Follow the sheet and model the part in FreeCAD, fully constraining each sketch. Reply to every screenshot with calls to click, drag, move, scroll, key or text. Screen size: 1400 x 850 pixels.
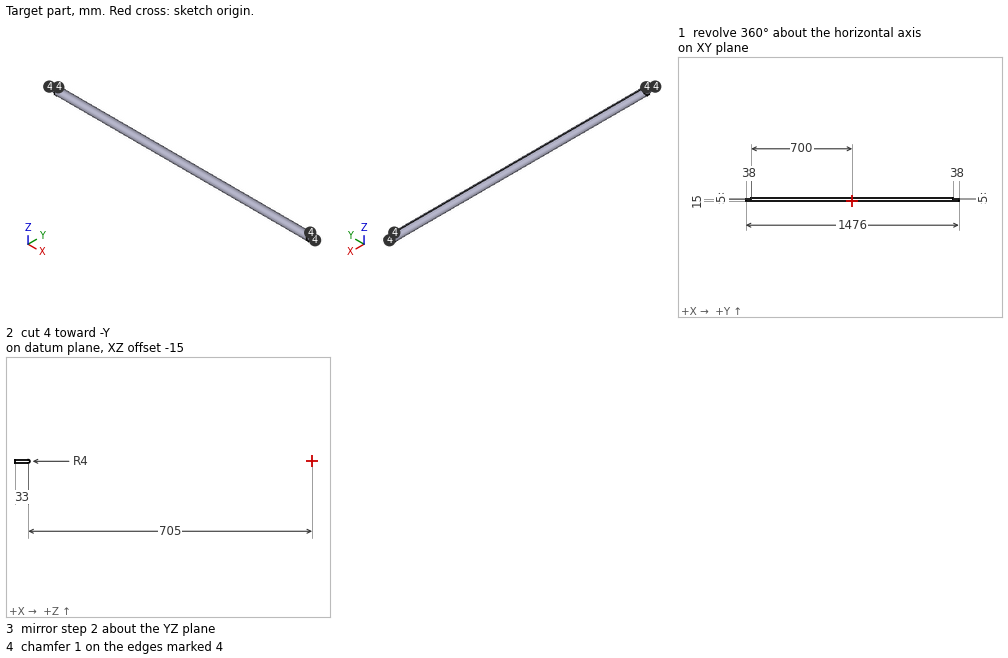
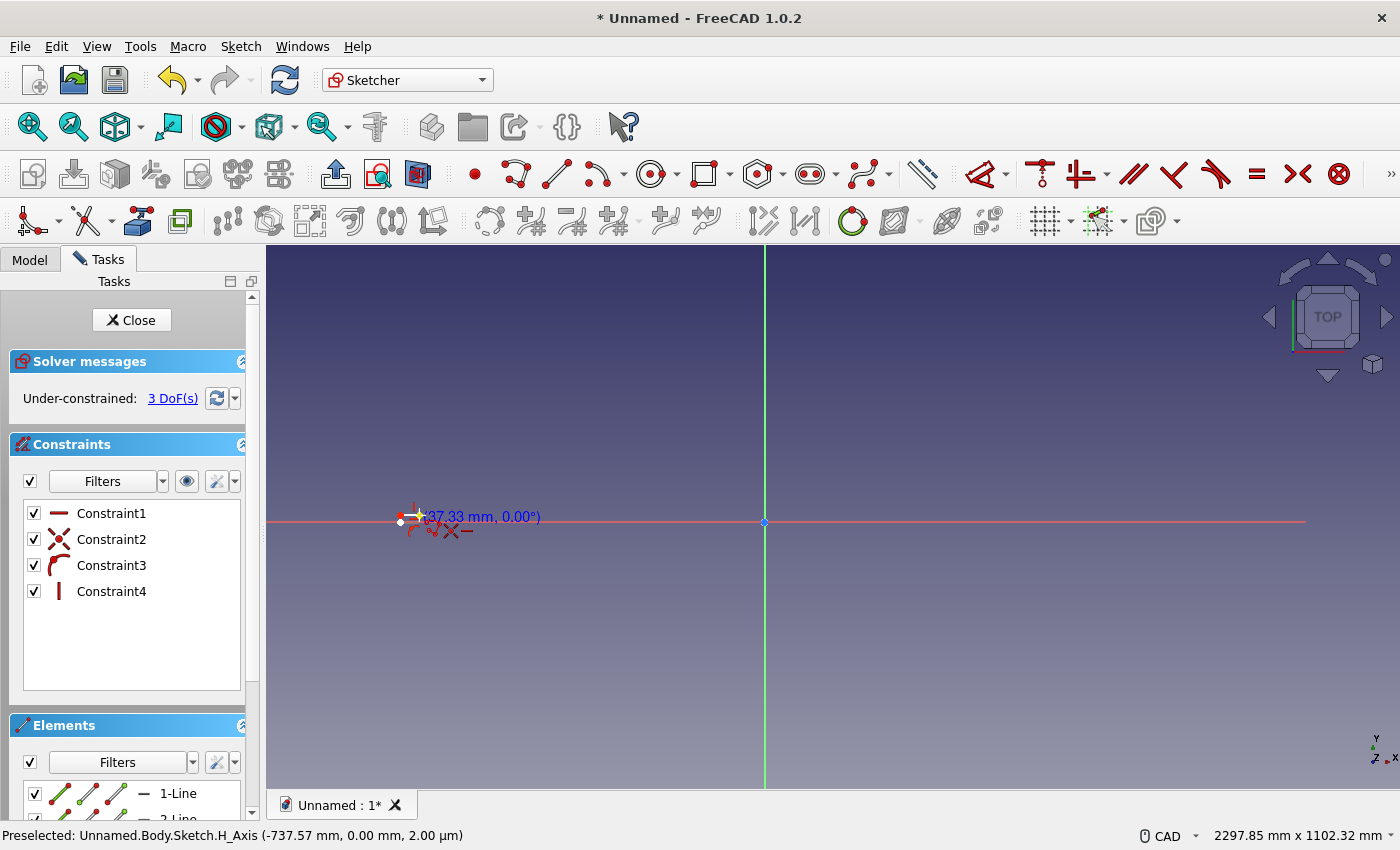
click(1129, 513)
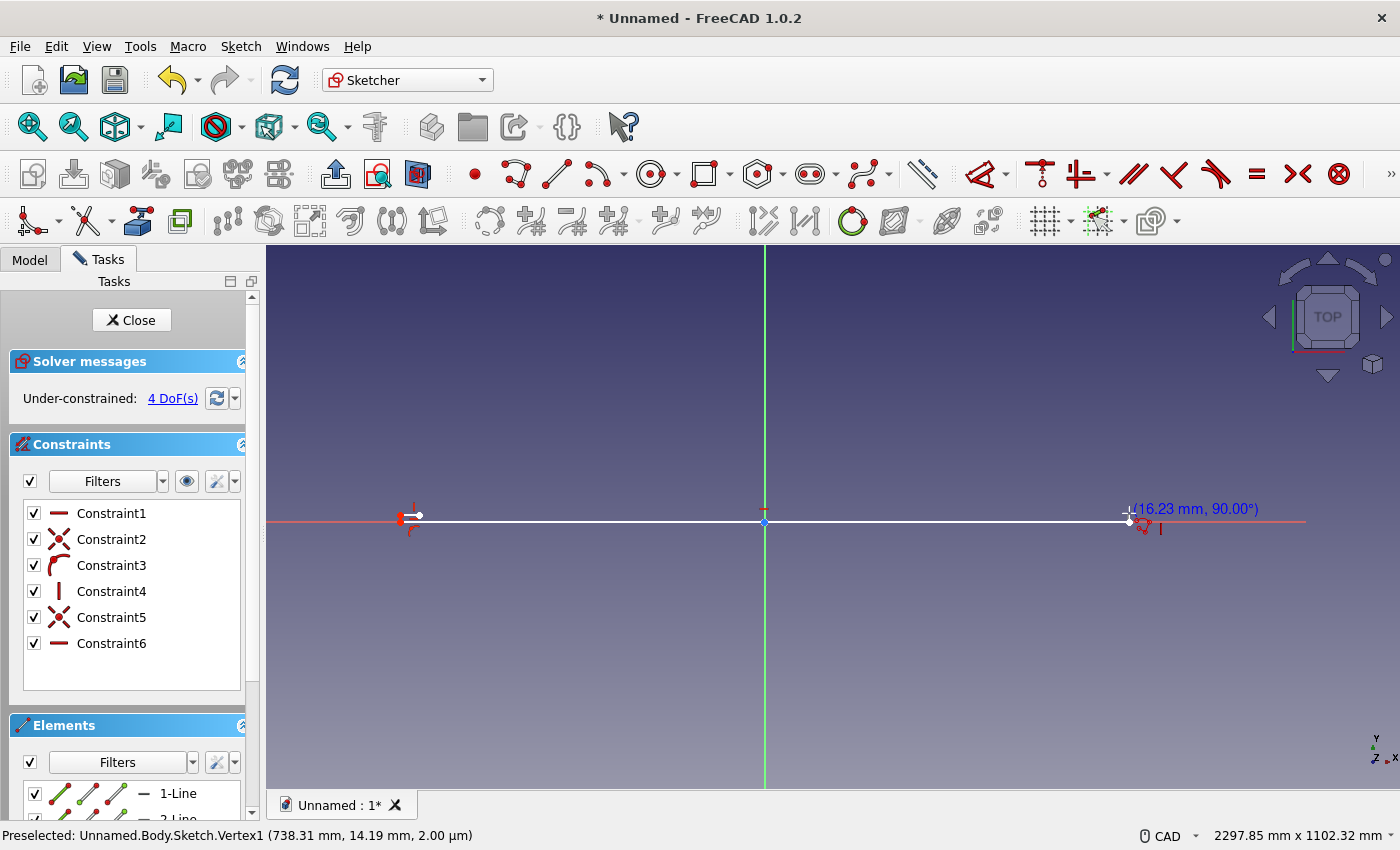
scroll(1129, 515, up, 4)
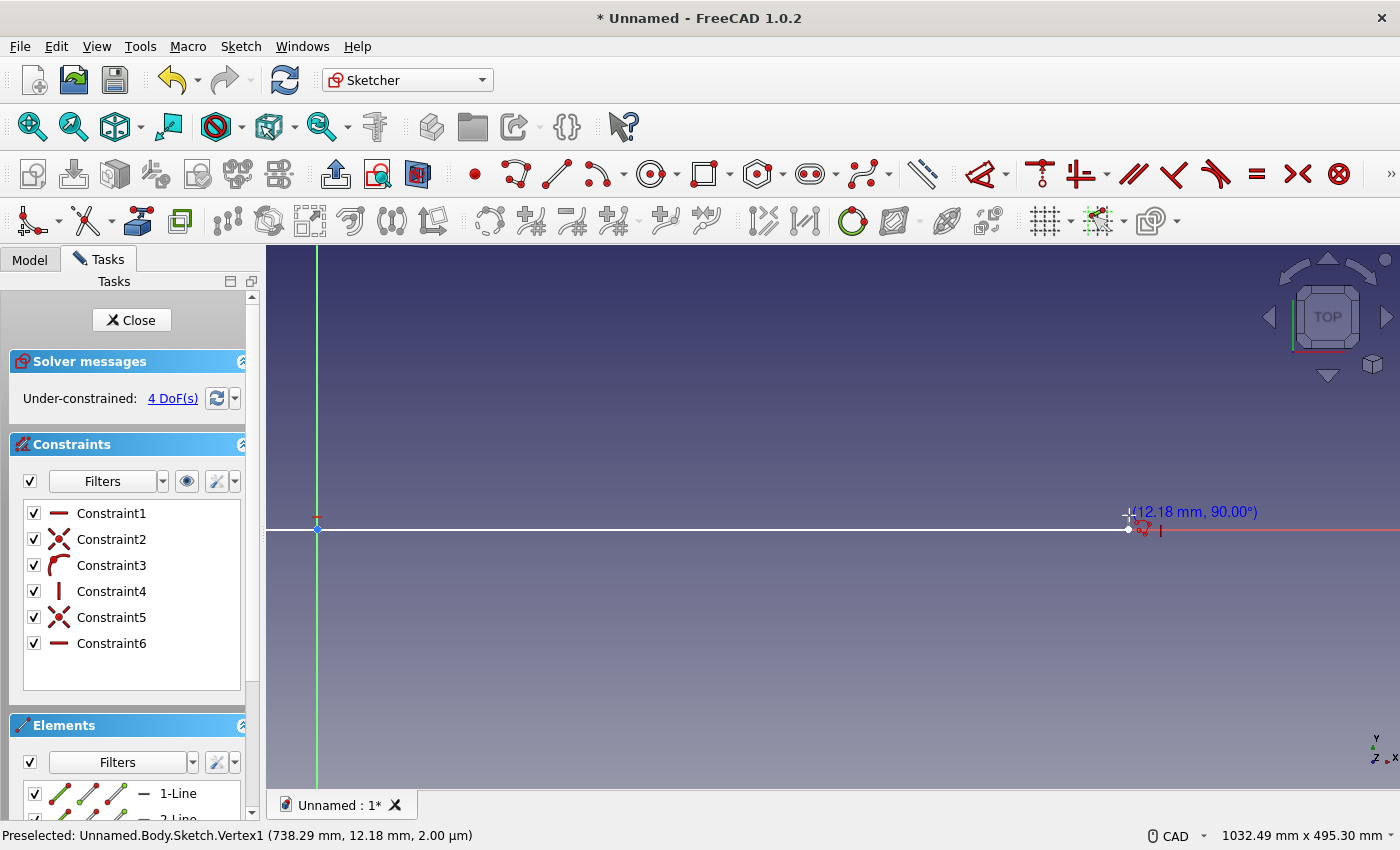
click(1128, 514)
click(1086, 514)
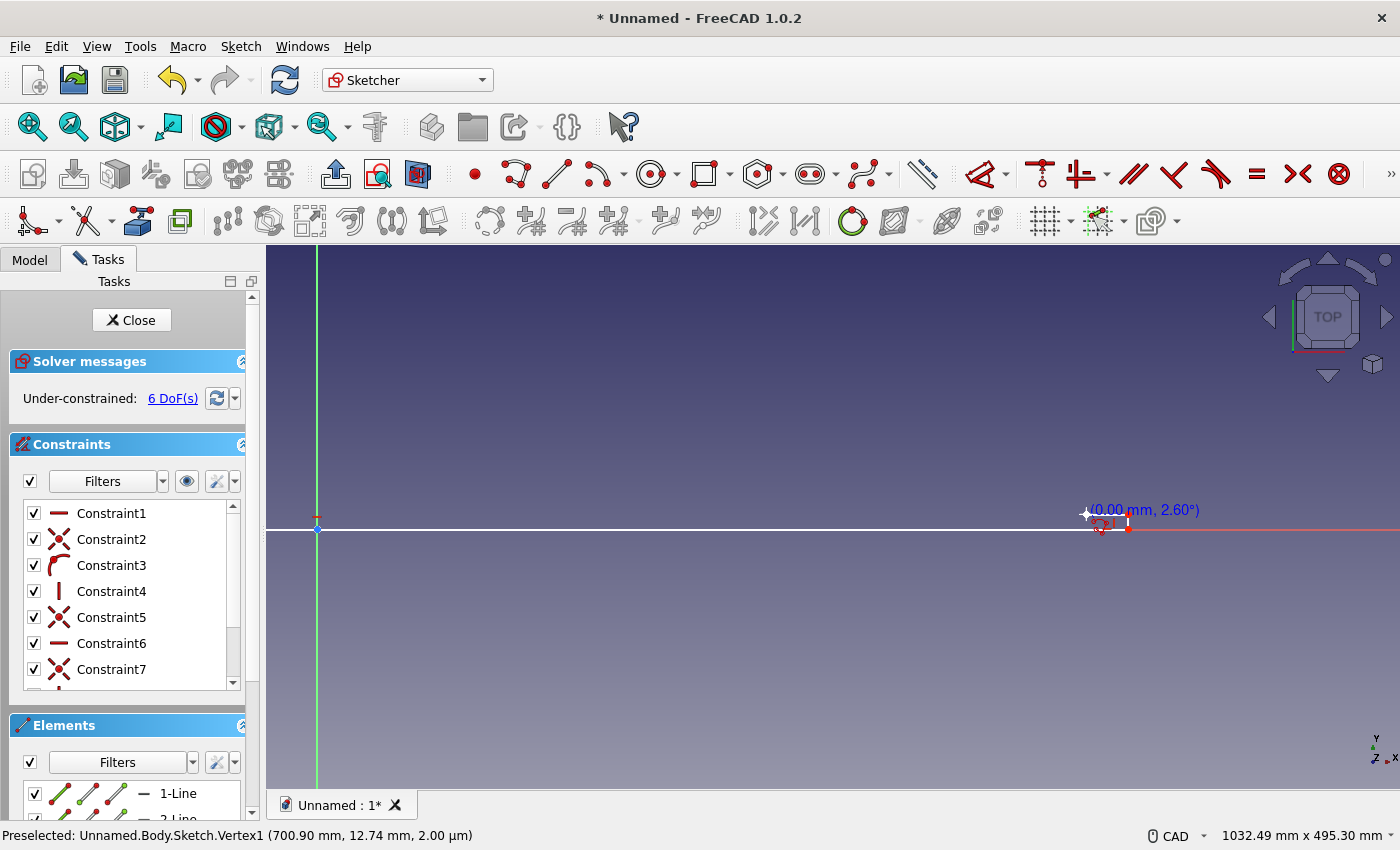
scroll(1086, 508, up, 6)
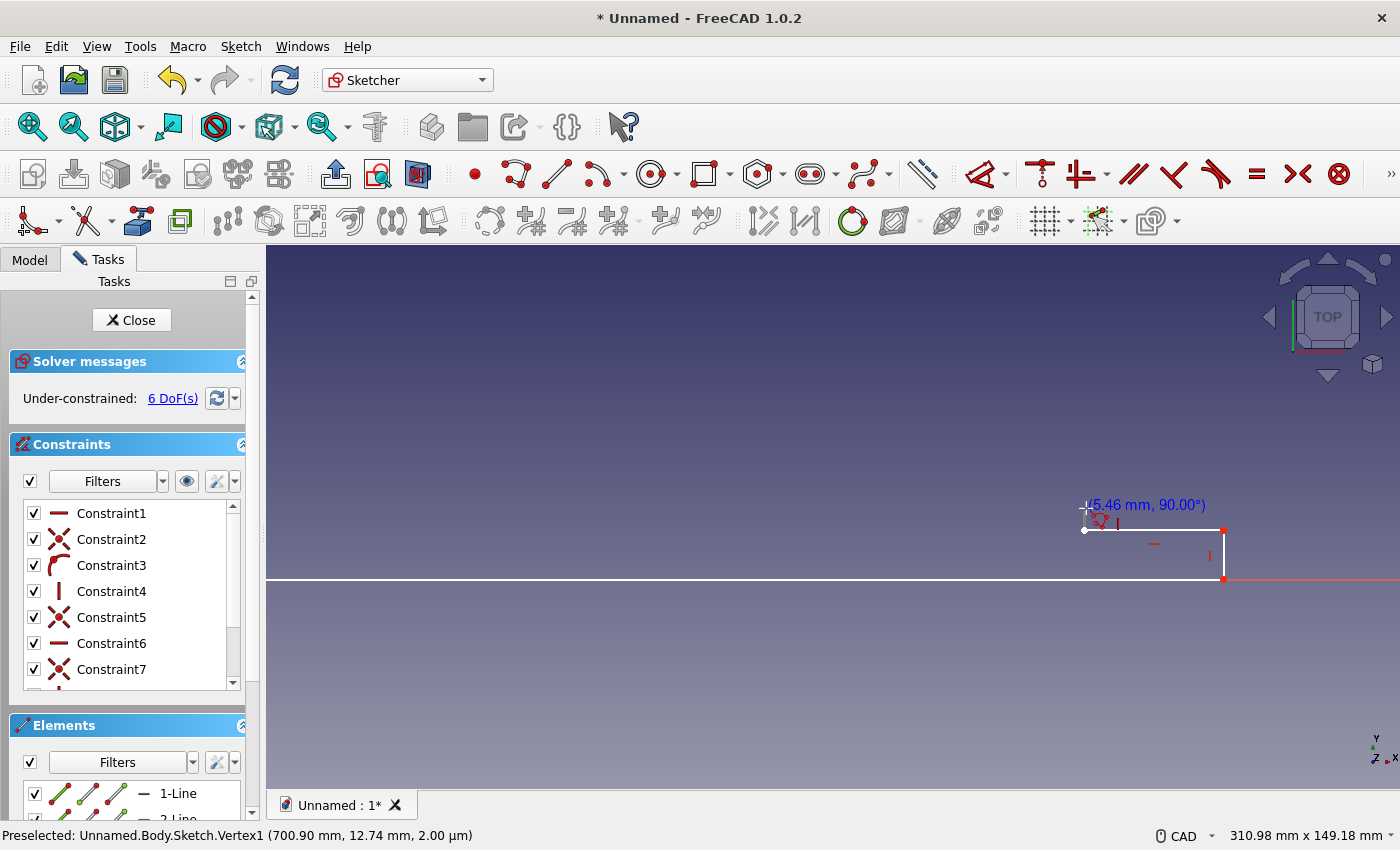
click(1084, 507)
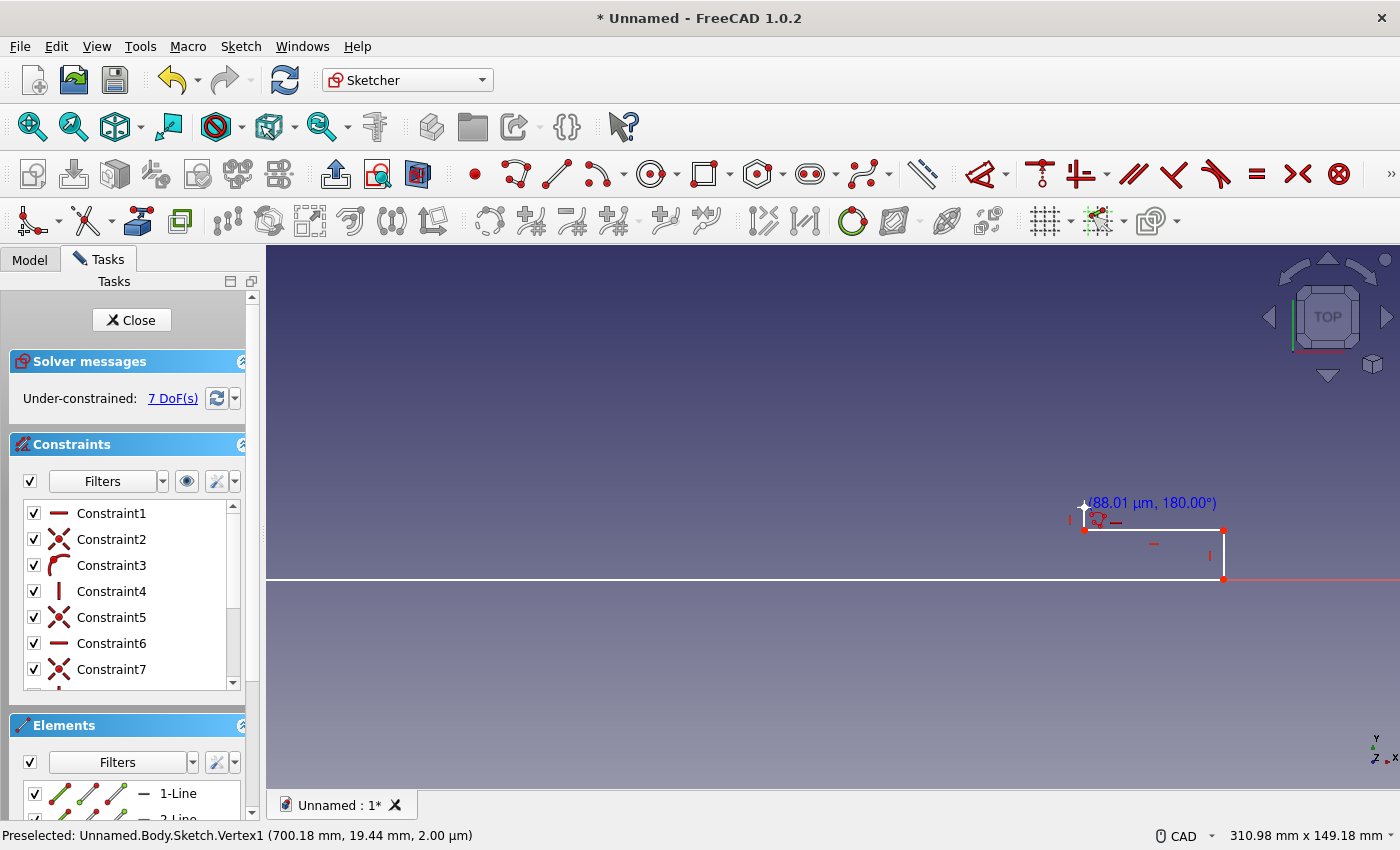
scroll(1114, 513, down, 10)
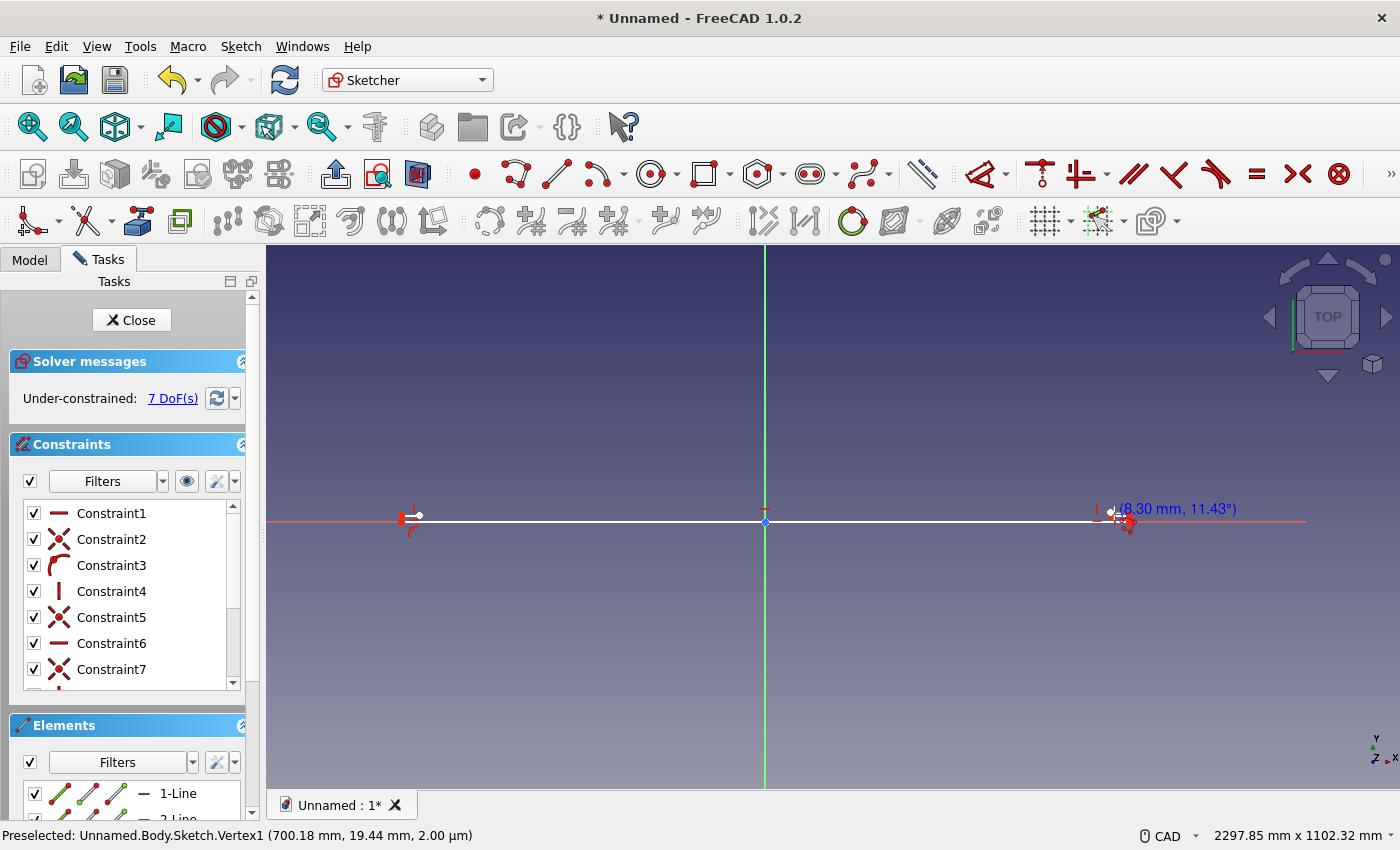
scroll(420, 513, up, 10)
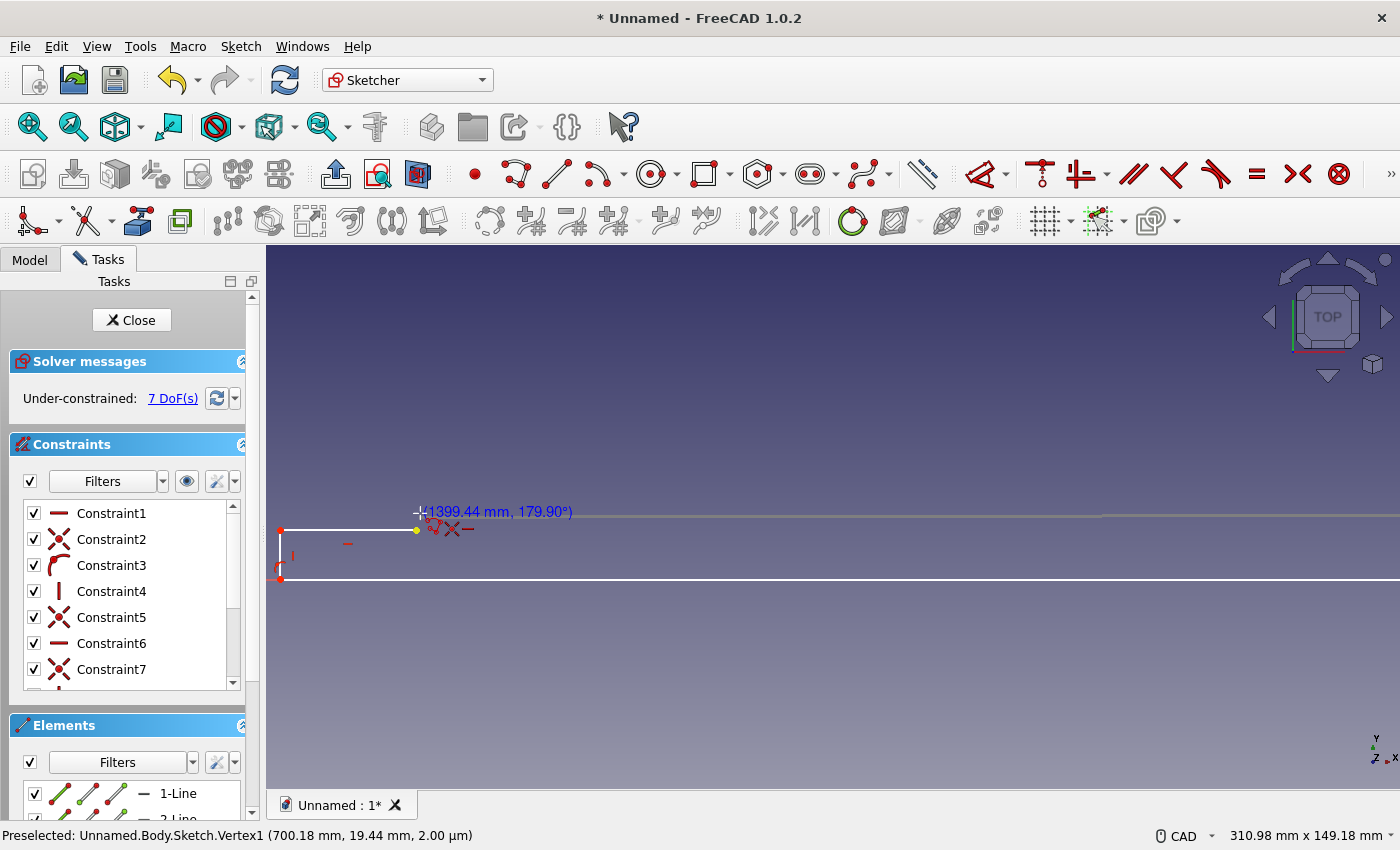
click(417, 507)
click(416, 530)
key(Escape)
key(Escape)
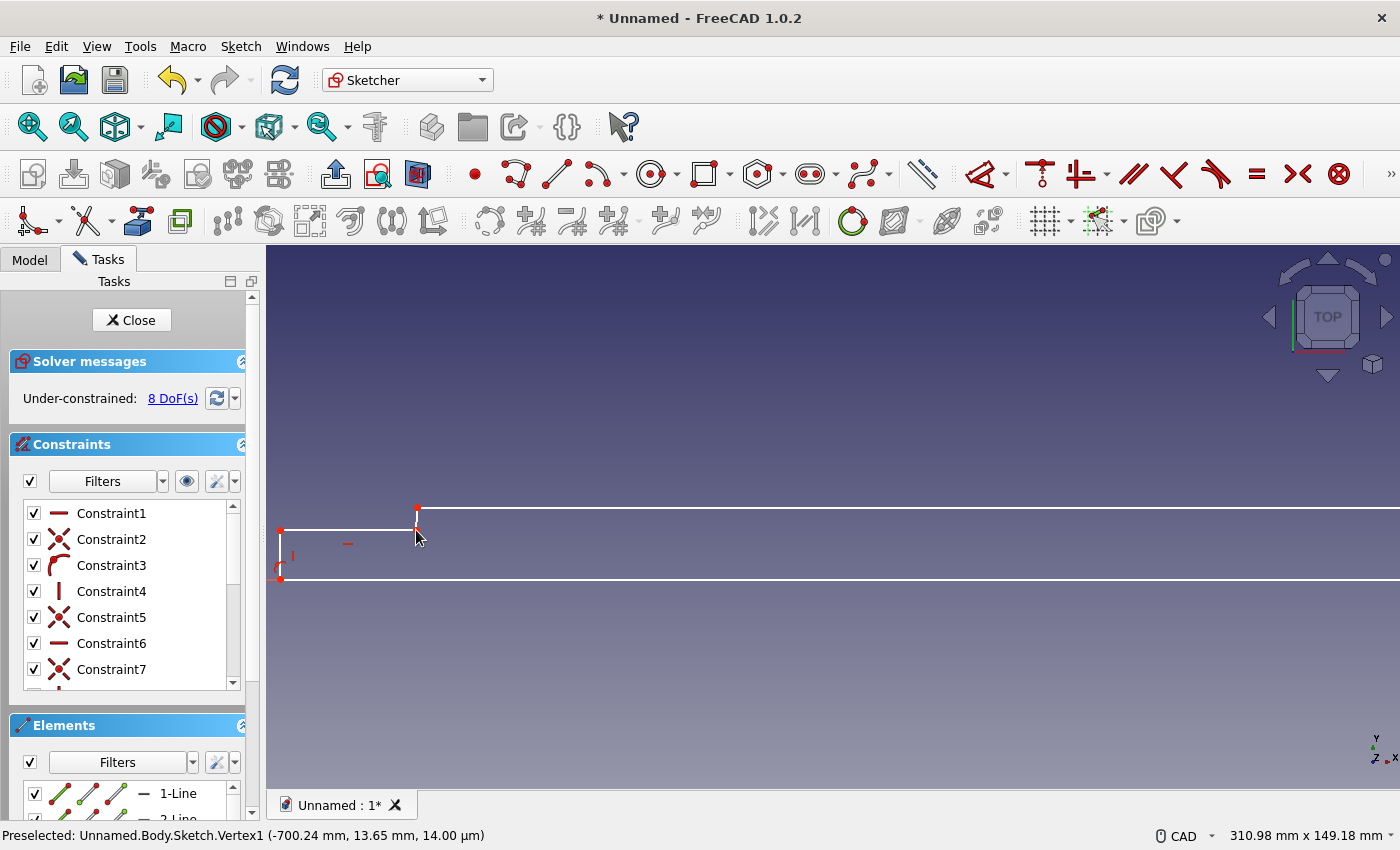
scroll(417, 519, up, 2)